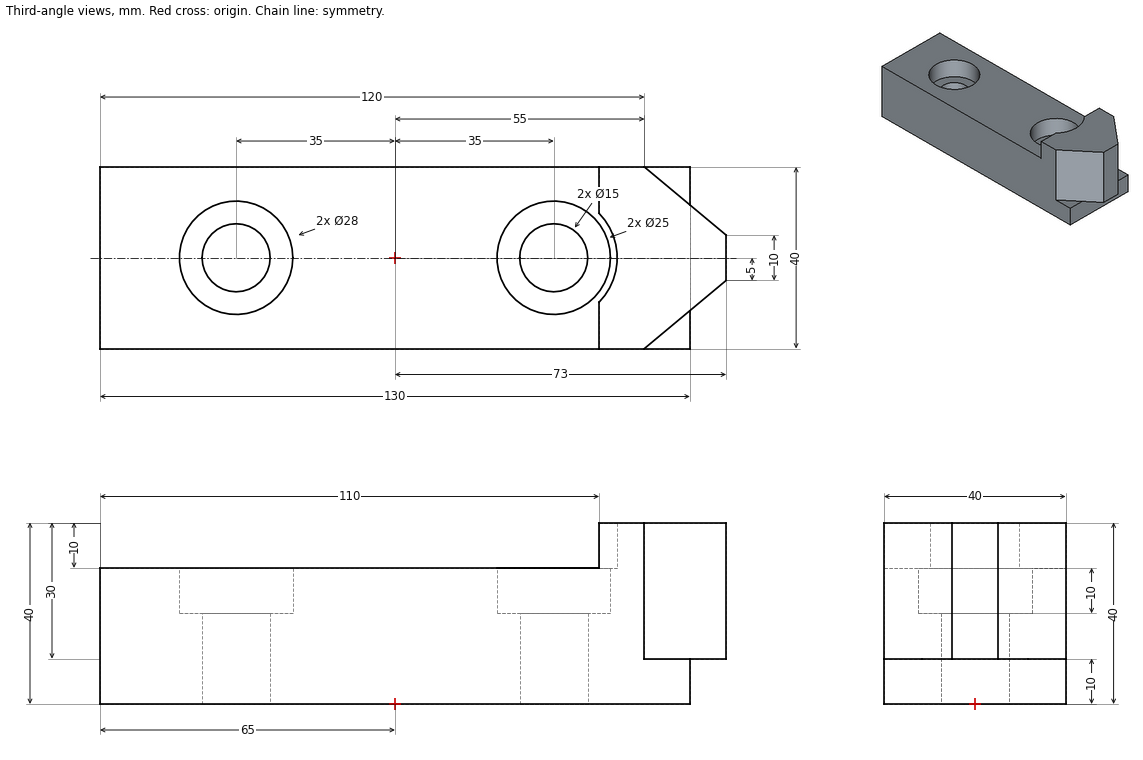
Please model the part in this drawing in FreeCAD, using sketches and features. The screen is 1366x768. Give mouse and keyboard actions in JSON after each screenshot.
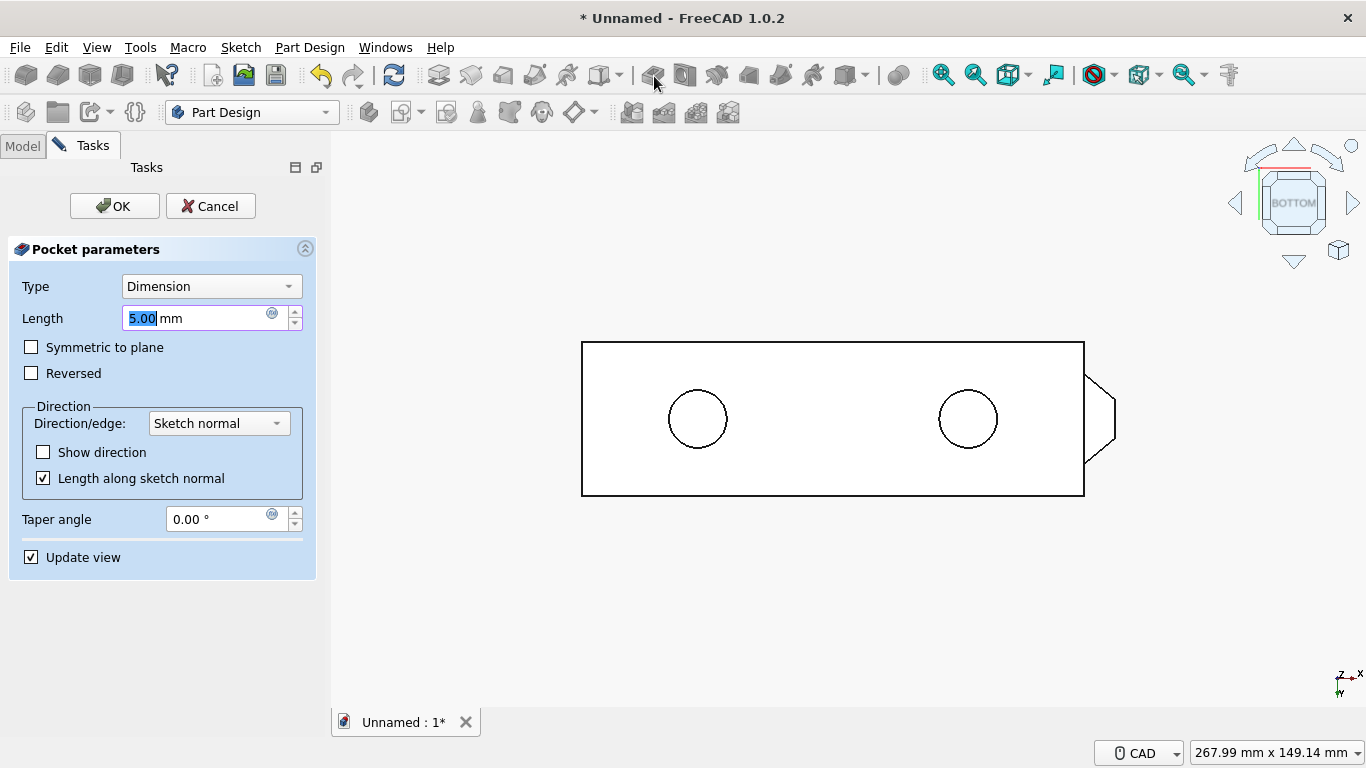
{"action": "type", "text": "40"}
{"action": "key", "text": "Tab"}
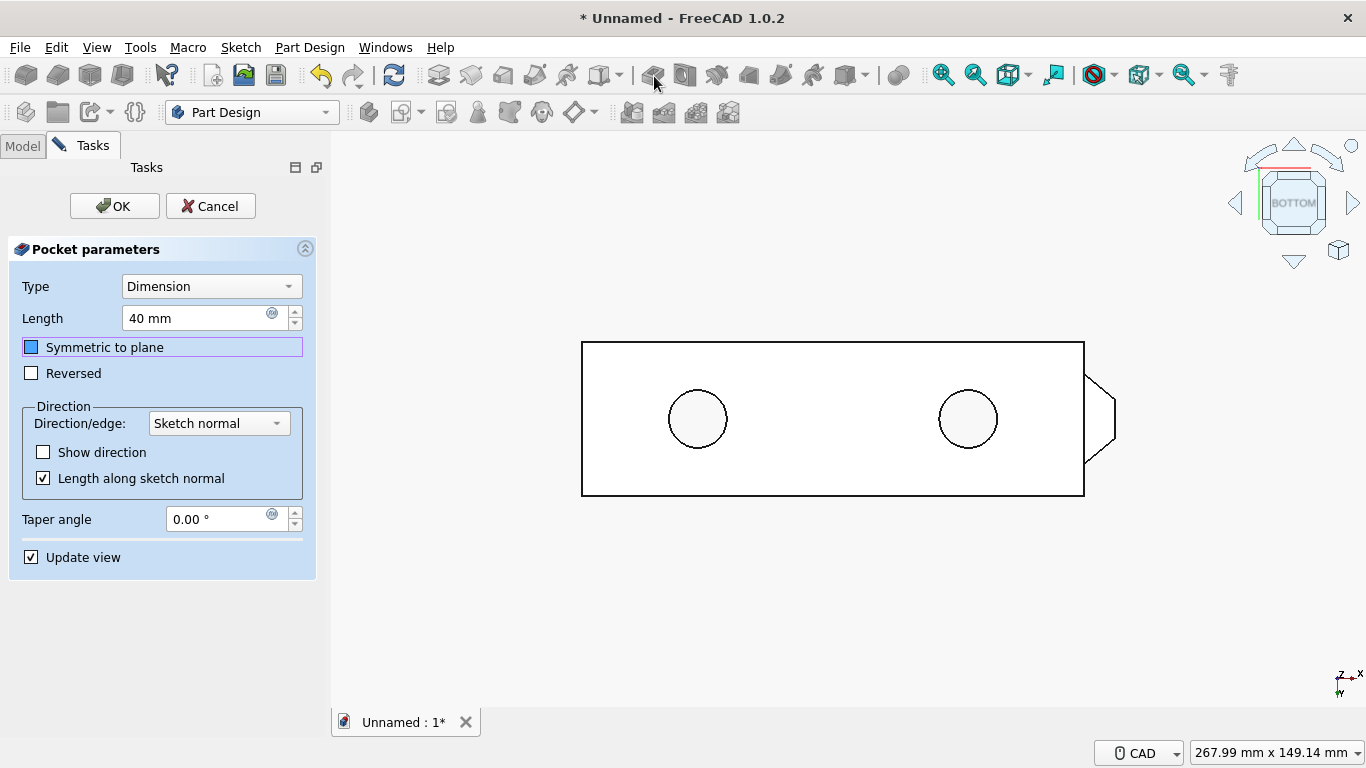
{"action": "left_click", "coordinate": [115, 206]}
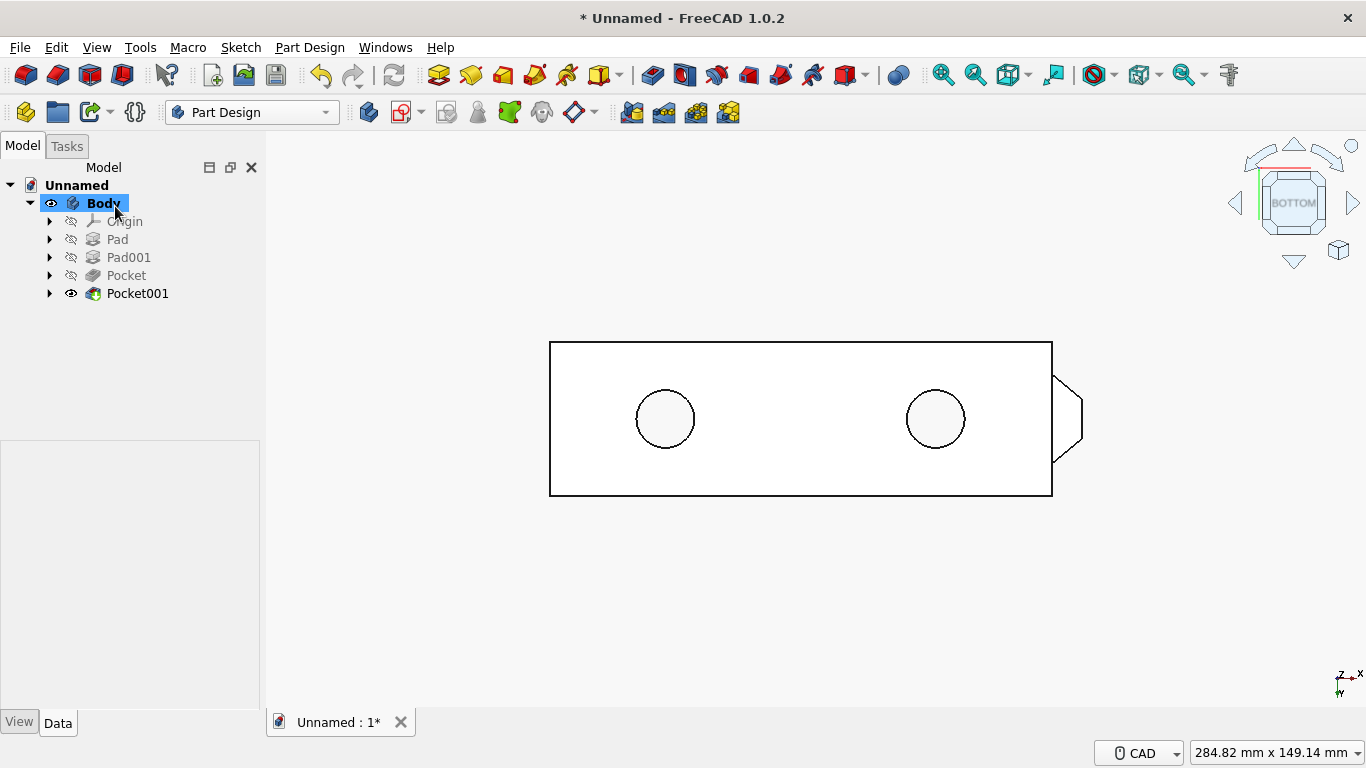
{"action": "key", "text": "0"}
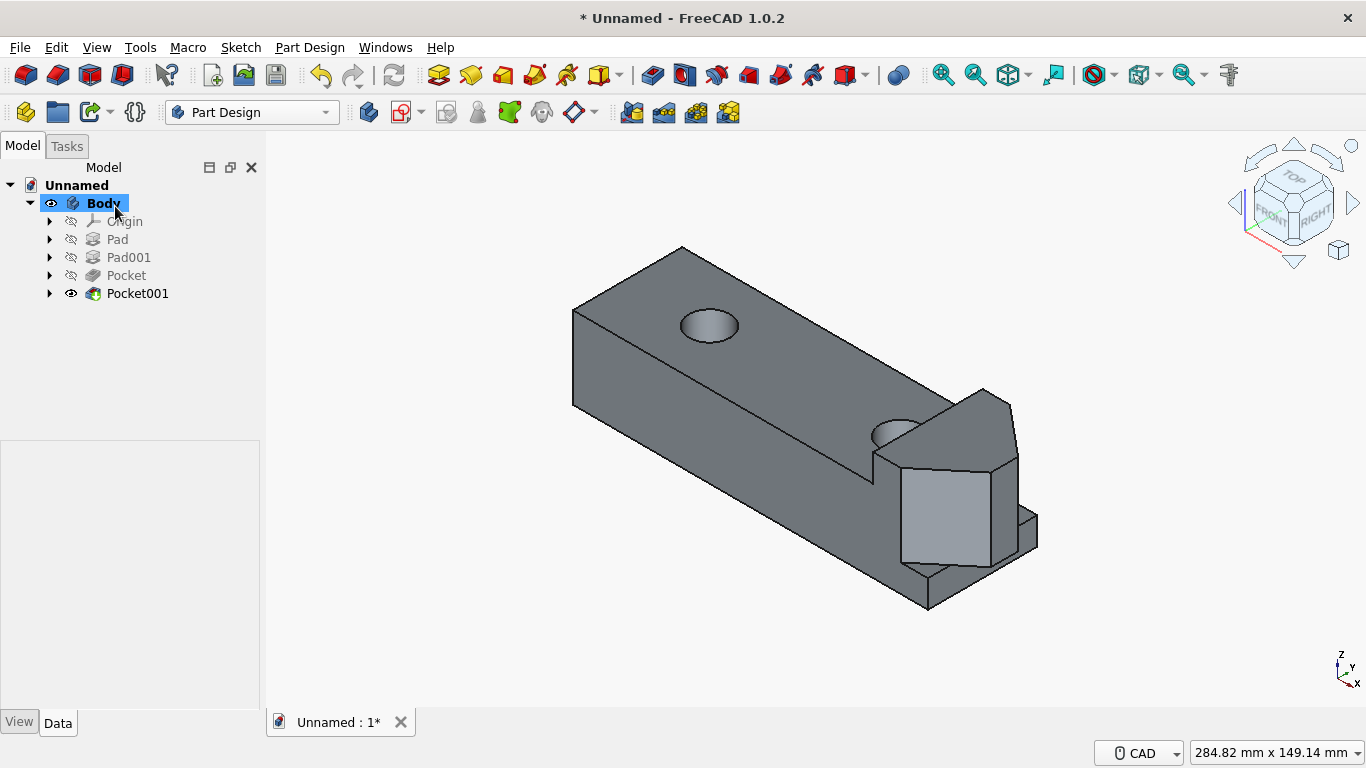
{"action": "left_click", "coordinate": [821, 389]}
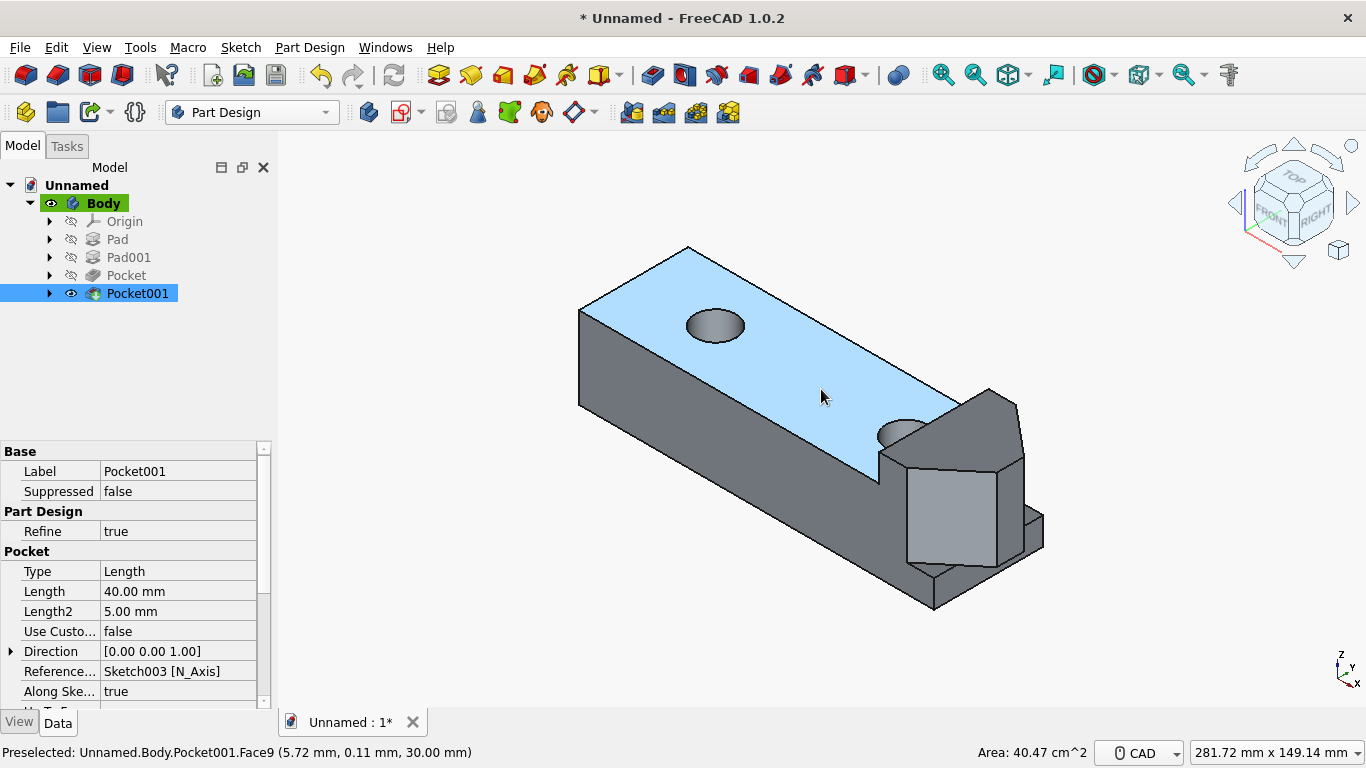
{"action": "left_click", "coordinate": [402, 112]}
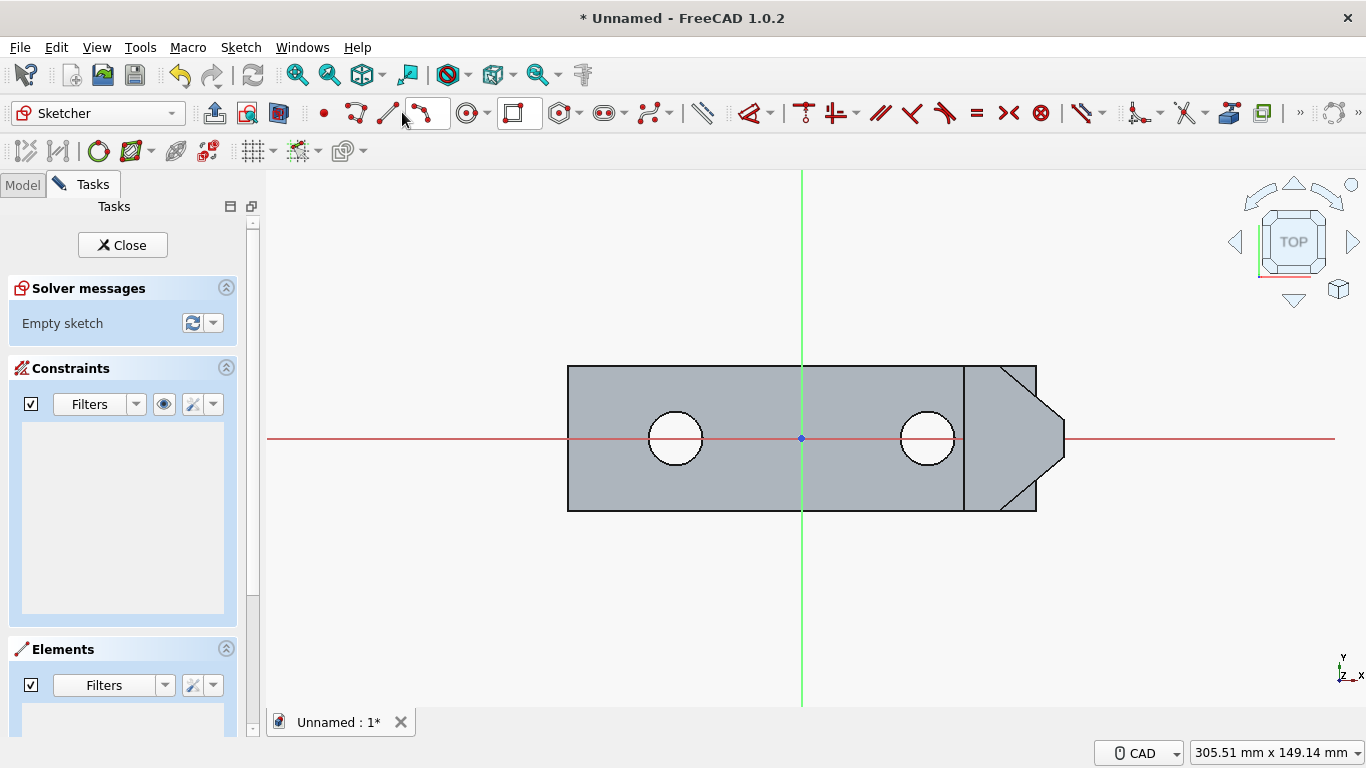
{"action": "left_click", "coordinate": [280, 114]}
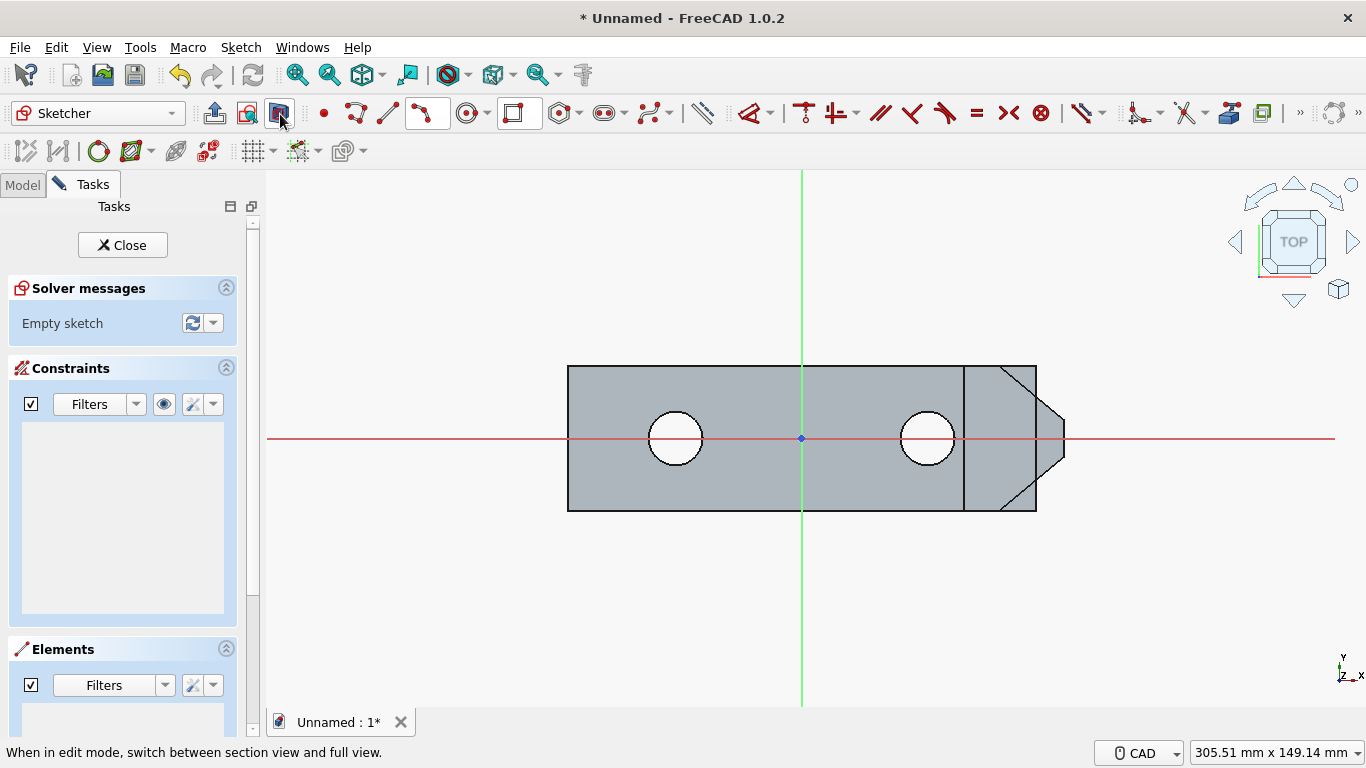
{"action": "scroll", "coordinate": [867, 438], "scroll_direction": "up", "scroll_amount": 3}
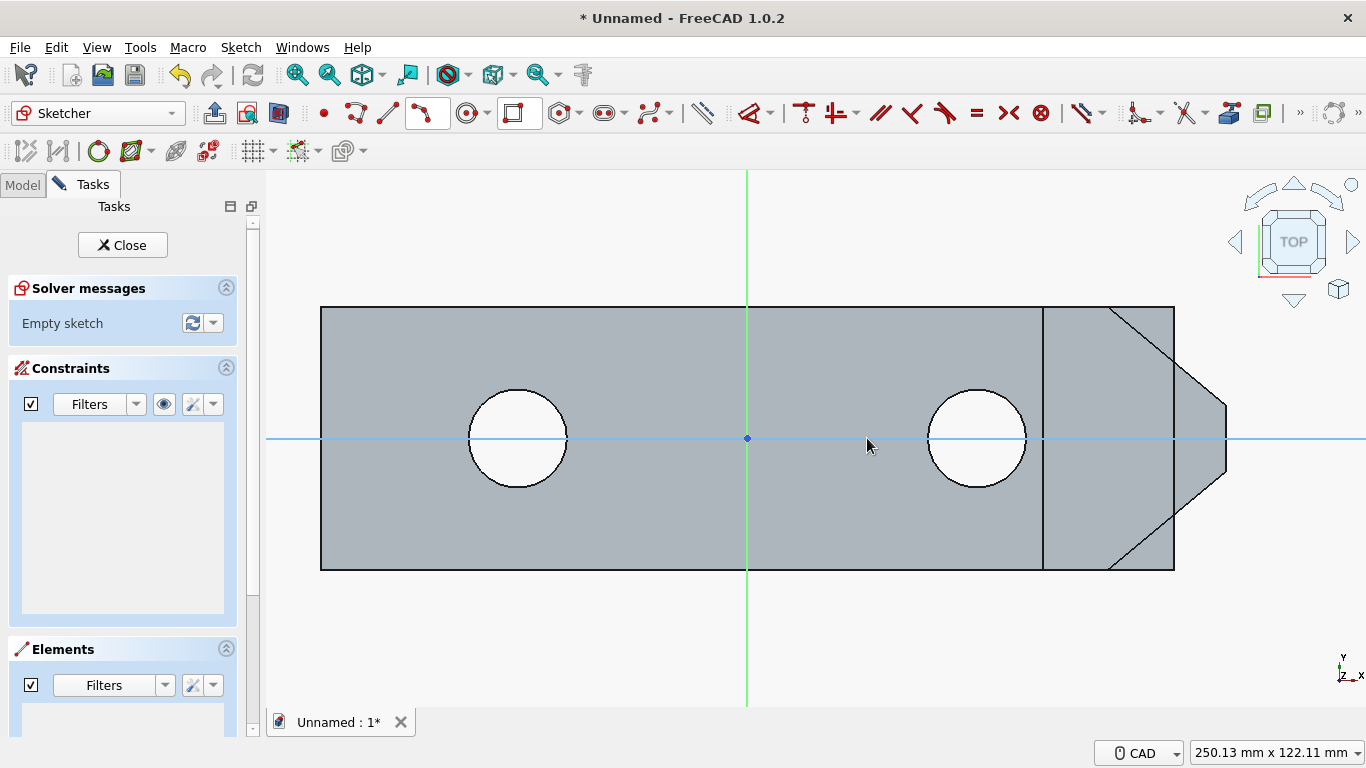
{"action": "left_click", "coordinate": [468, 114]}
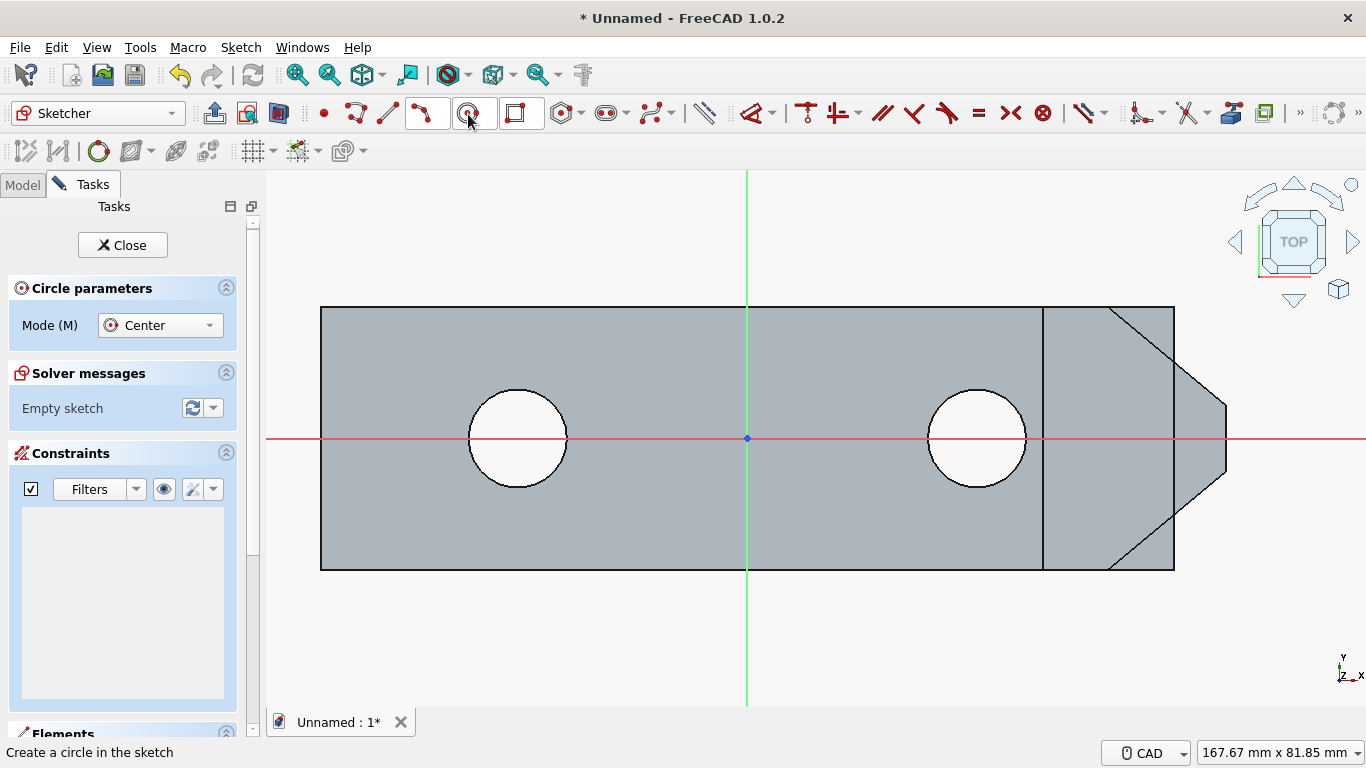
{"action": "left_click", "coordinate": [518, 438]}
{"action": "left_click", "coordinate": [583, 374]}